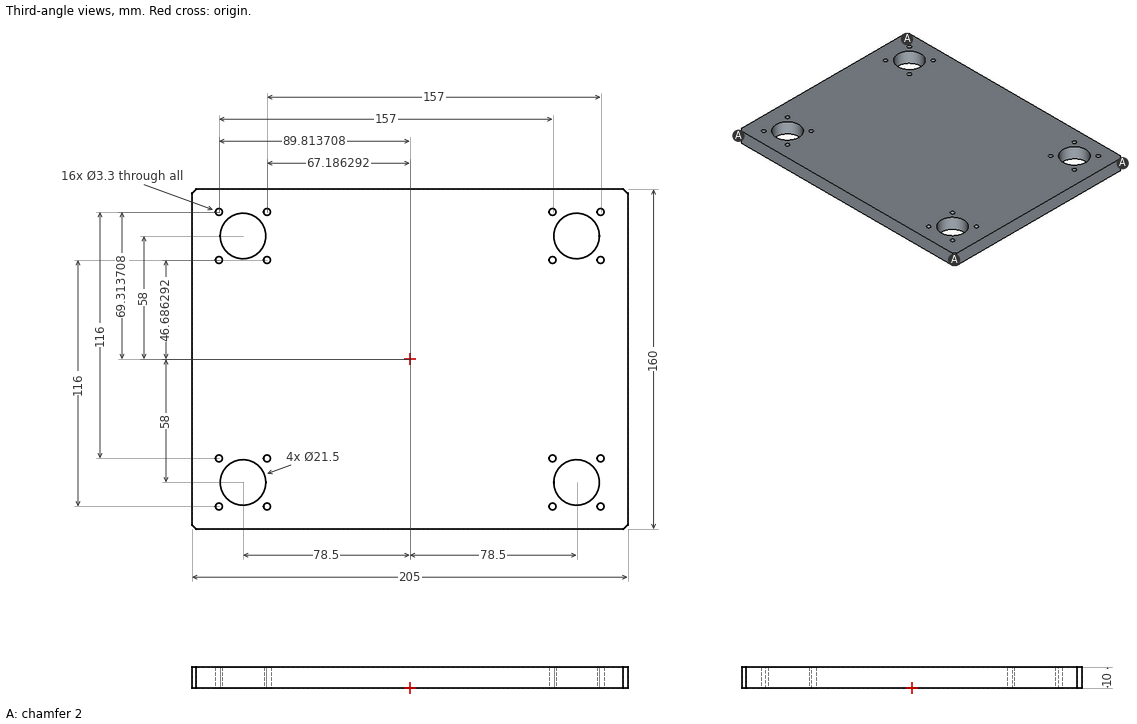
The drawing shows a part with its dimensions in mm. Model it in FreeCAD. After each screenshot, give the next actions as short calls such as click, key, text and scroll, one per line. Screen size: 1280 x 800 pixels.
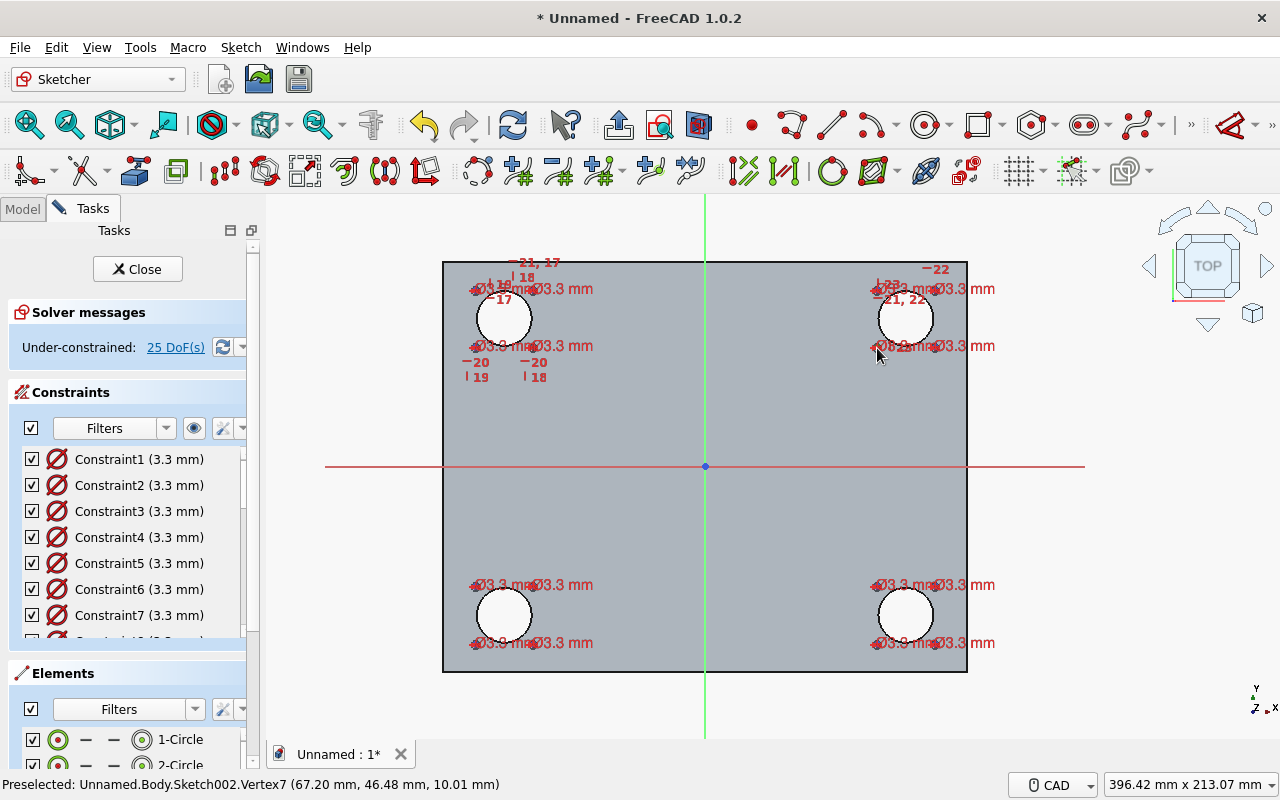
key(h)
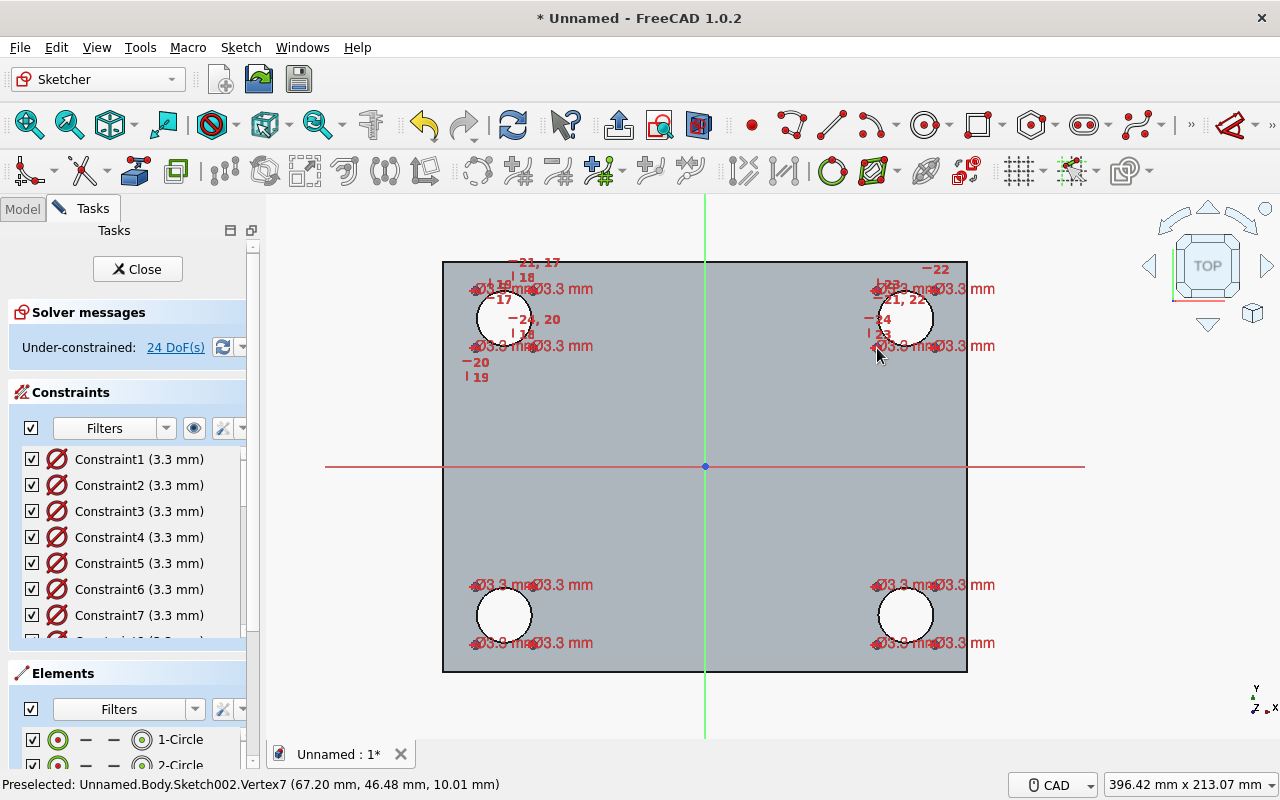
click(935, 291)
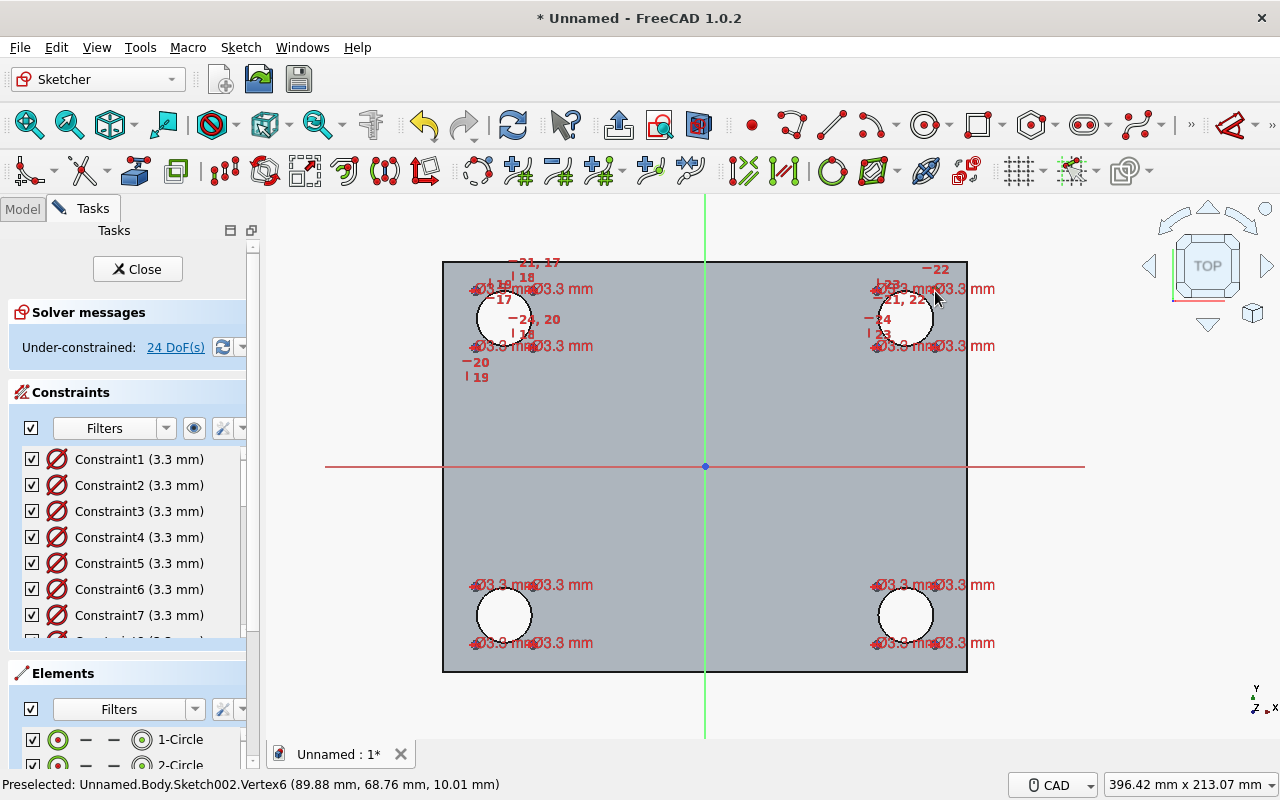
click(935, 348)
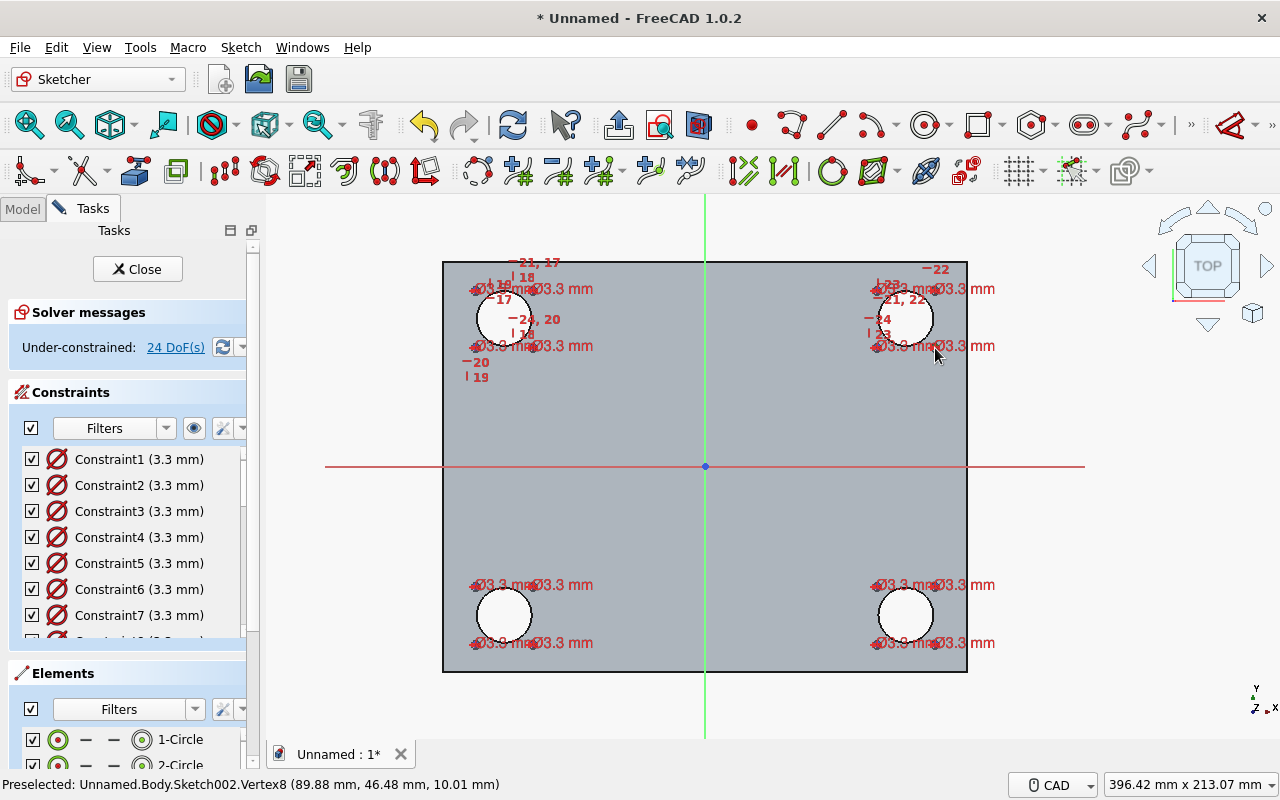
key(v)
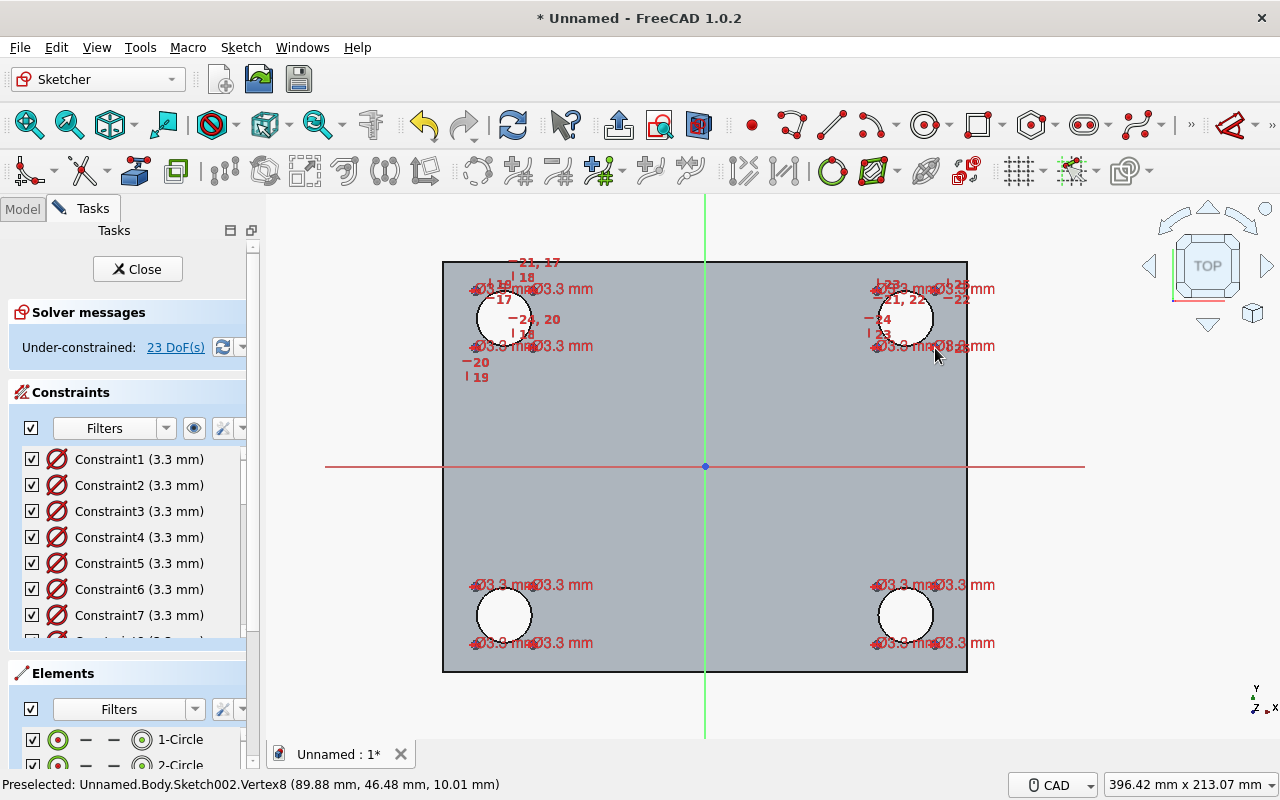
click(877, 348)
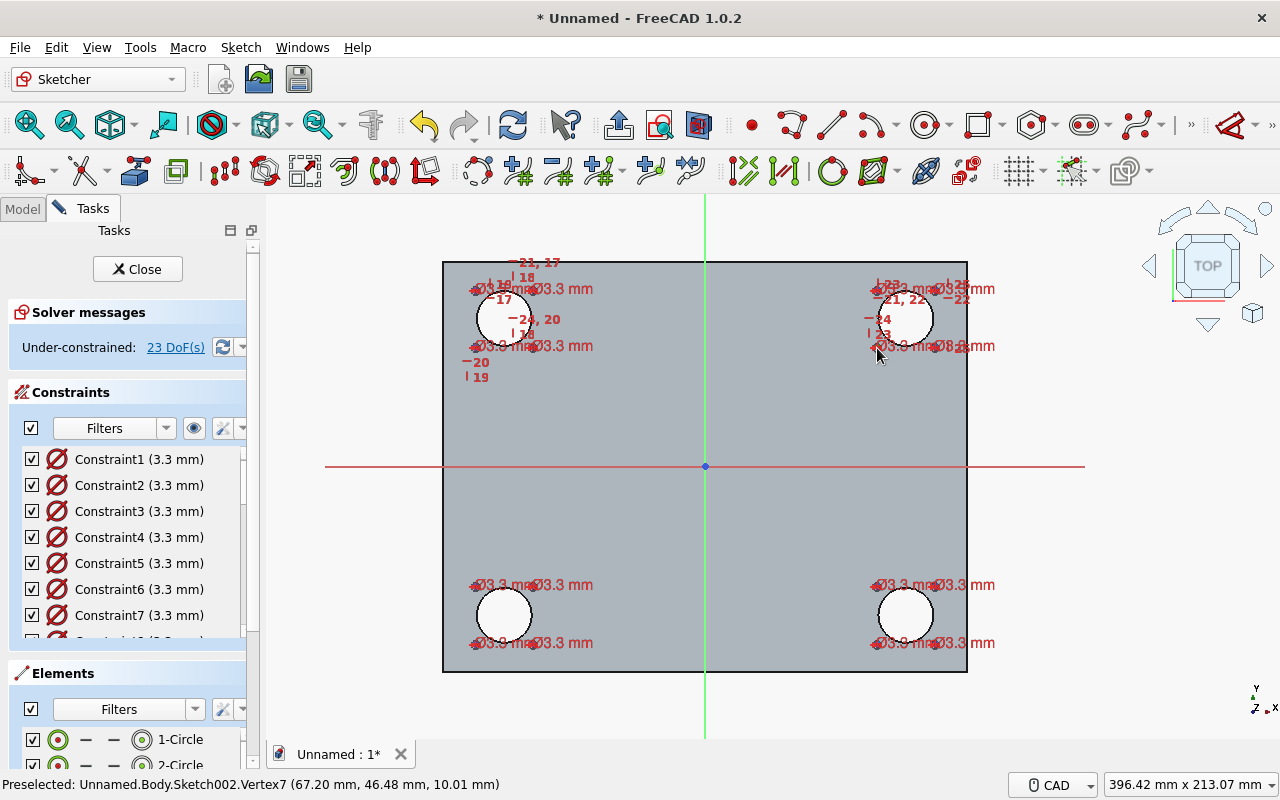
click(935, 348)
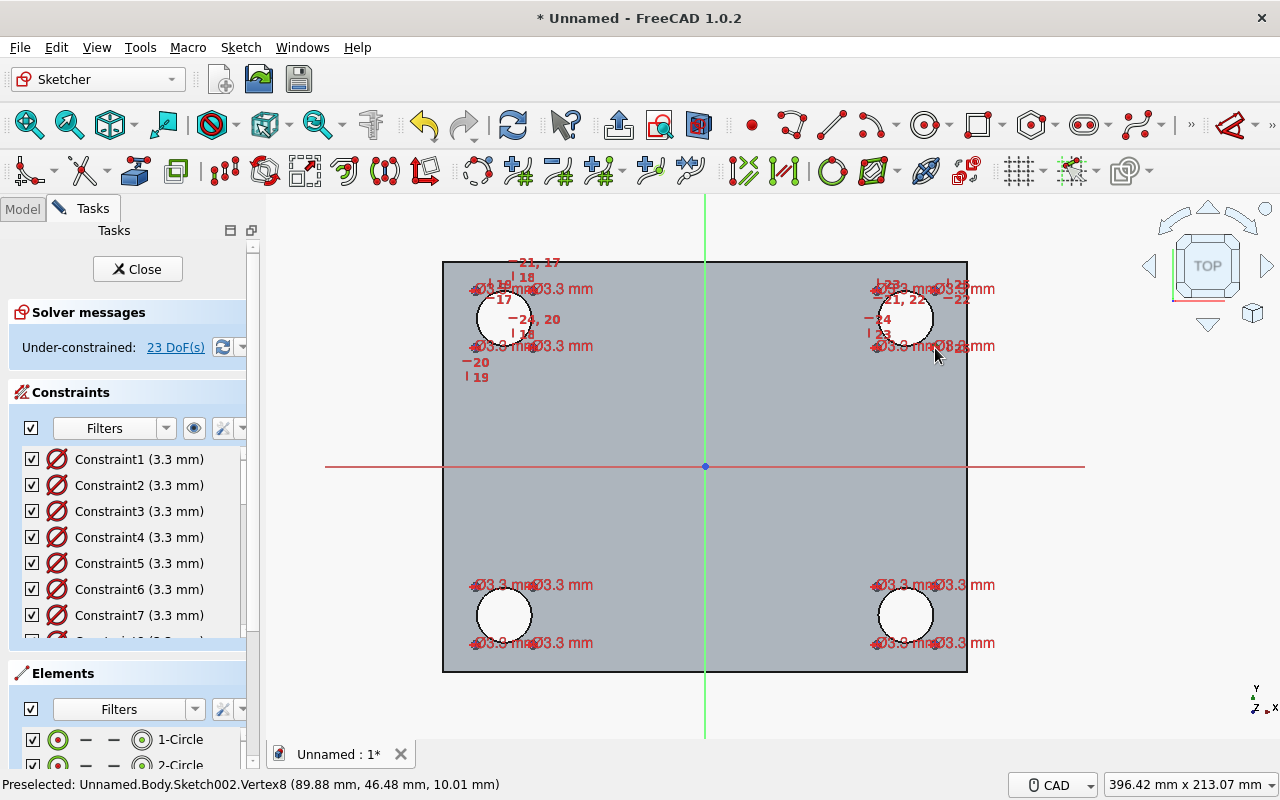
key(h)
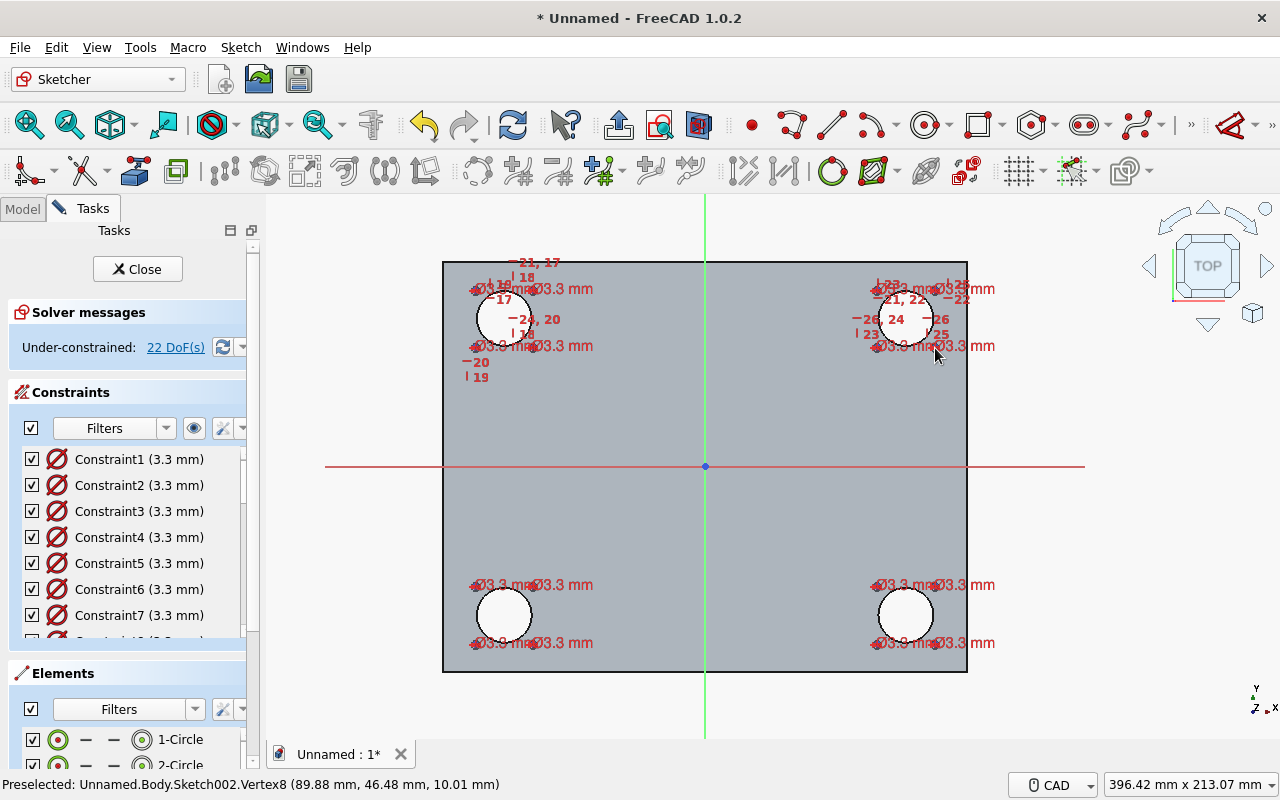
click(476, 348)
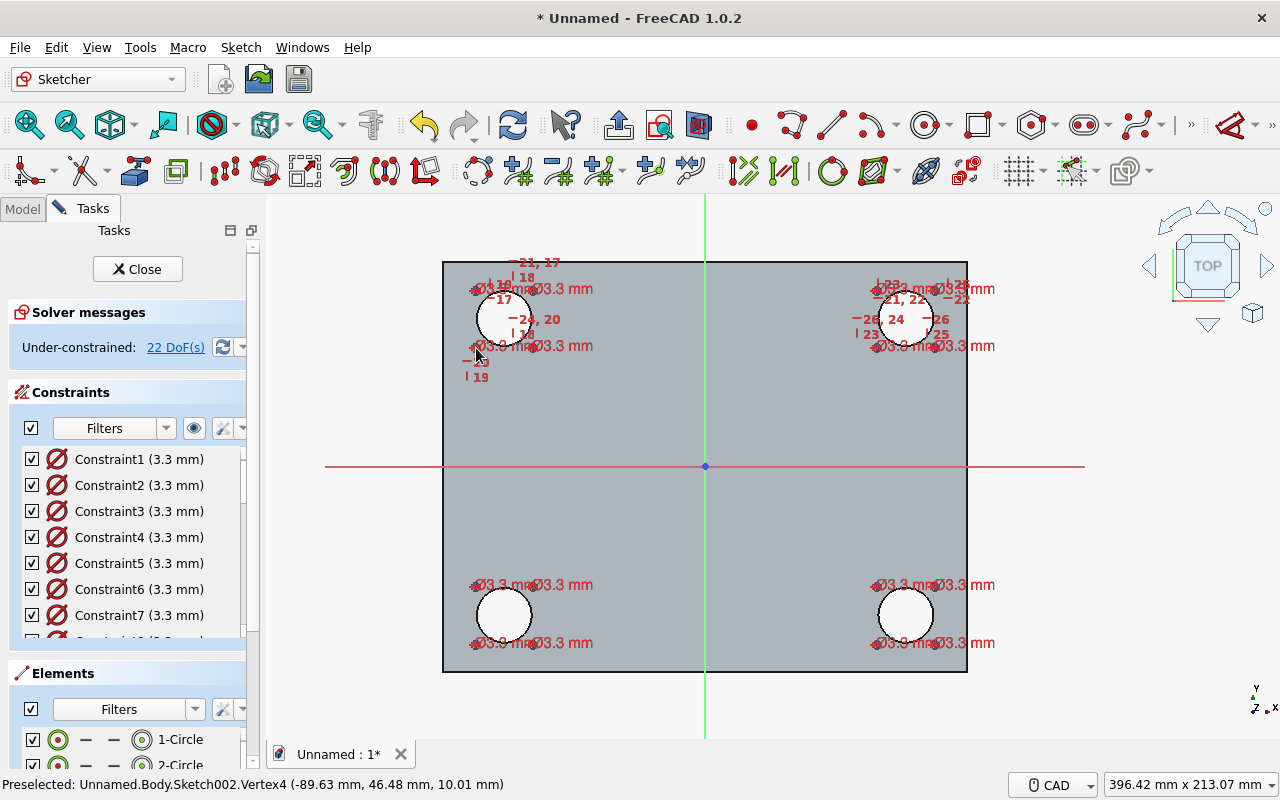
click(476, 587)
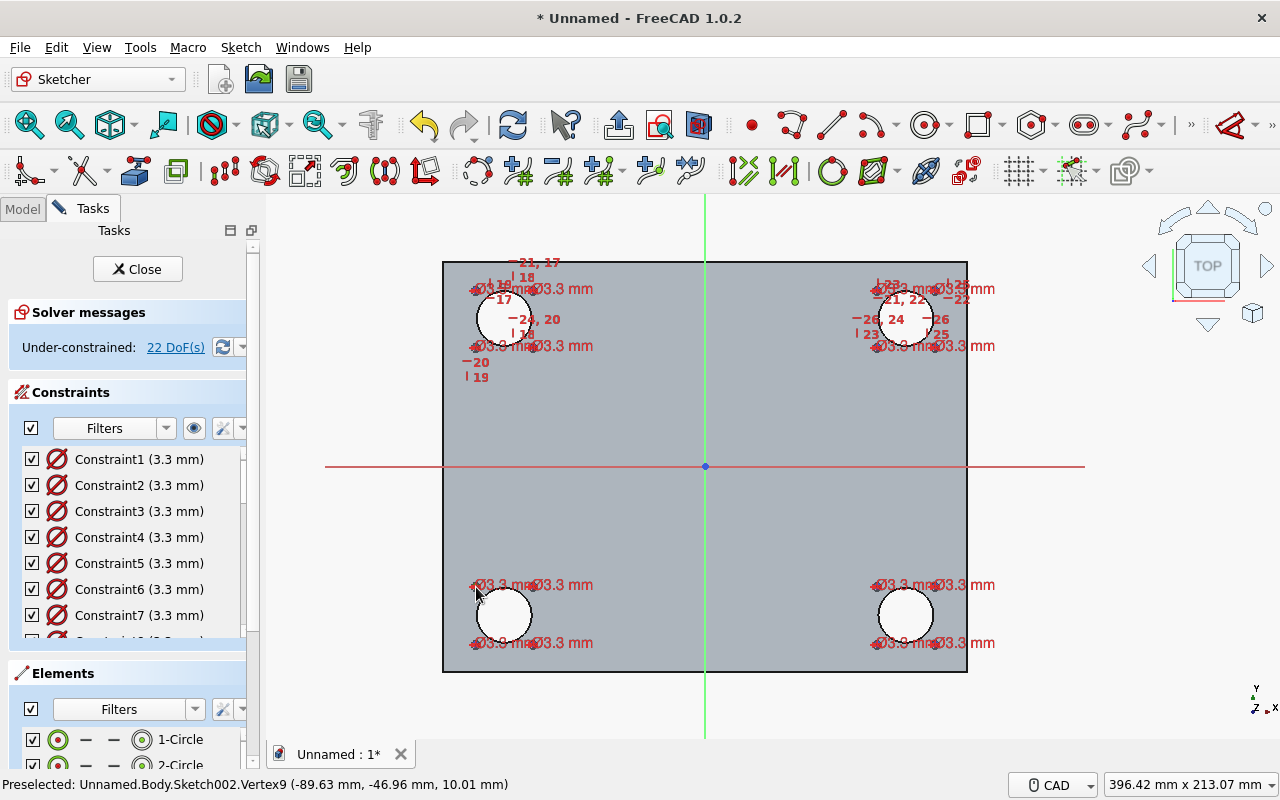
key(v)